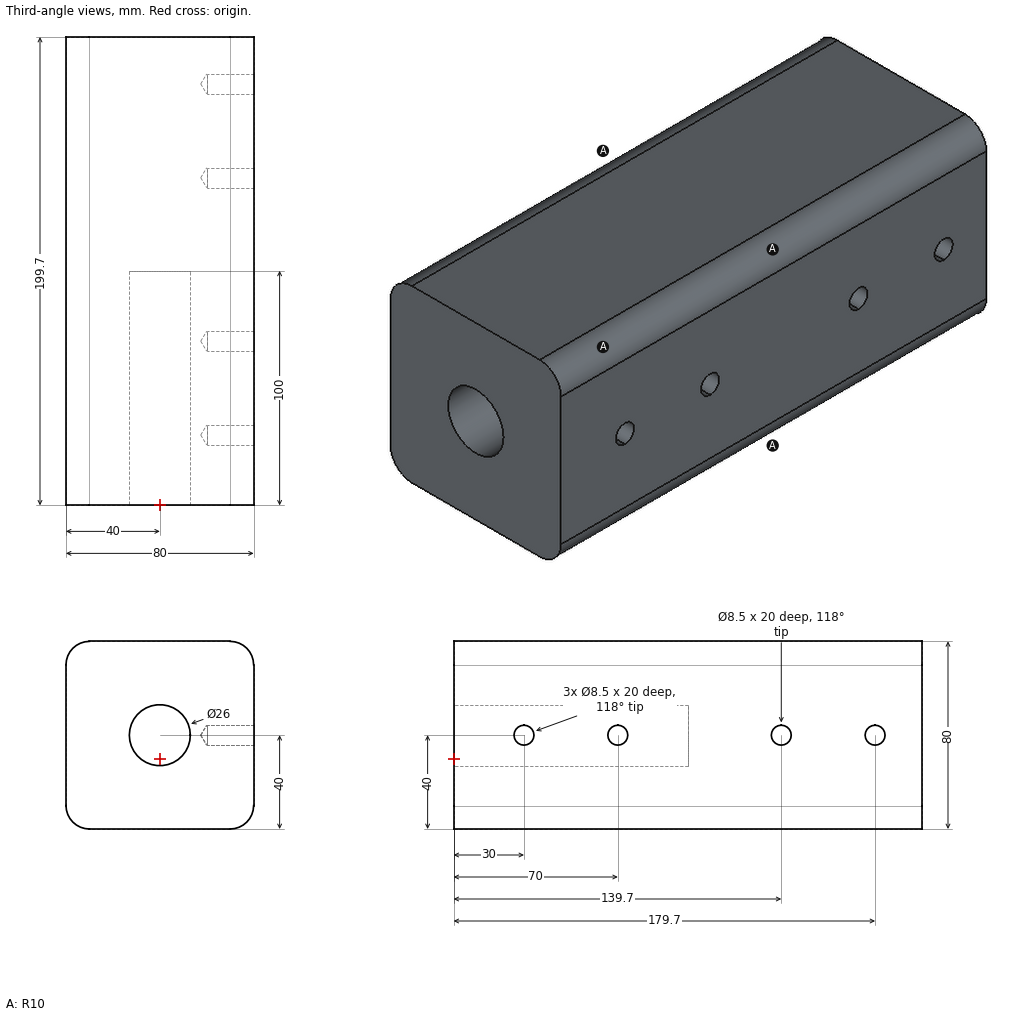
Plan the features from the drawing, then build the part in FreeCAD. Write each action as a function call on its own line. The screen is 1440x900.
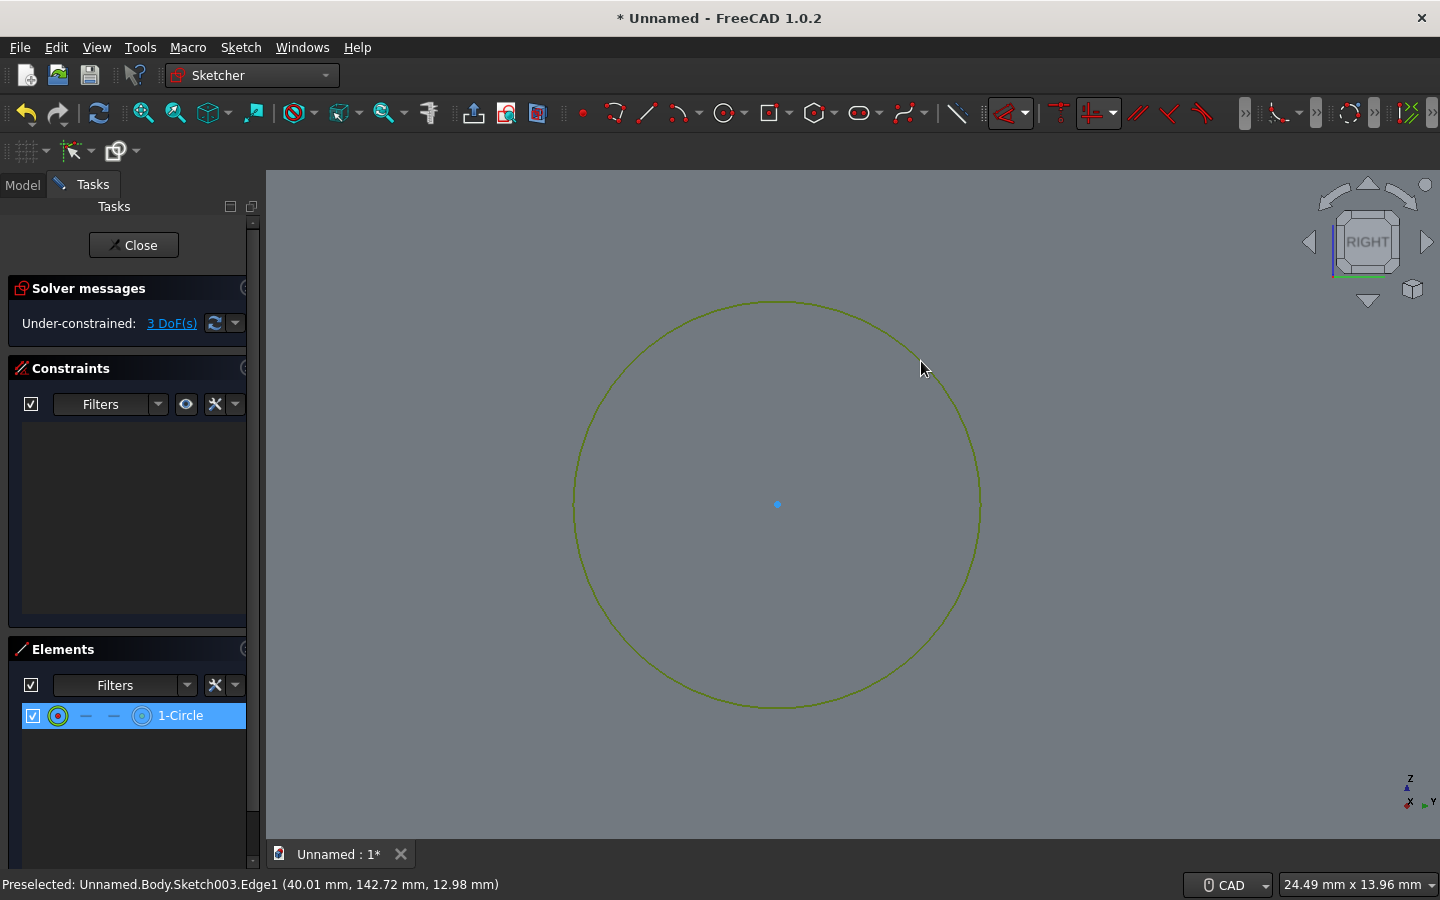
key(k)
key(o)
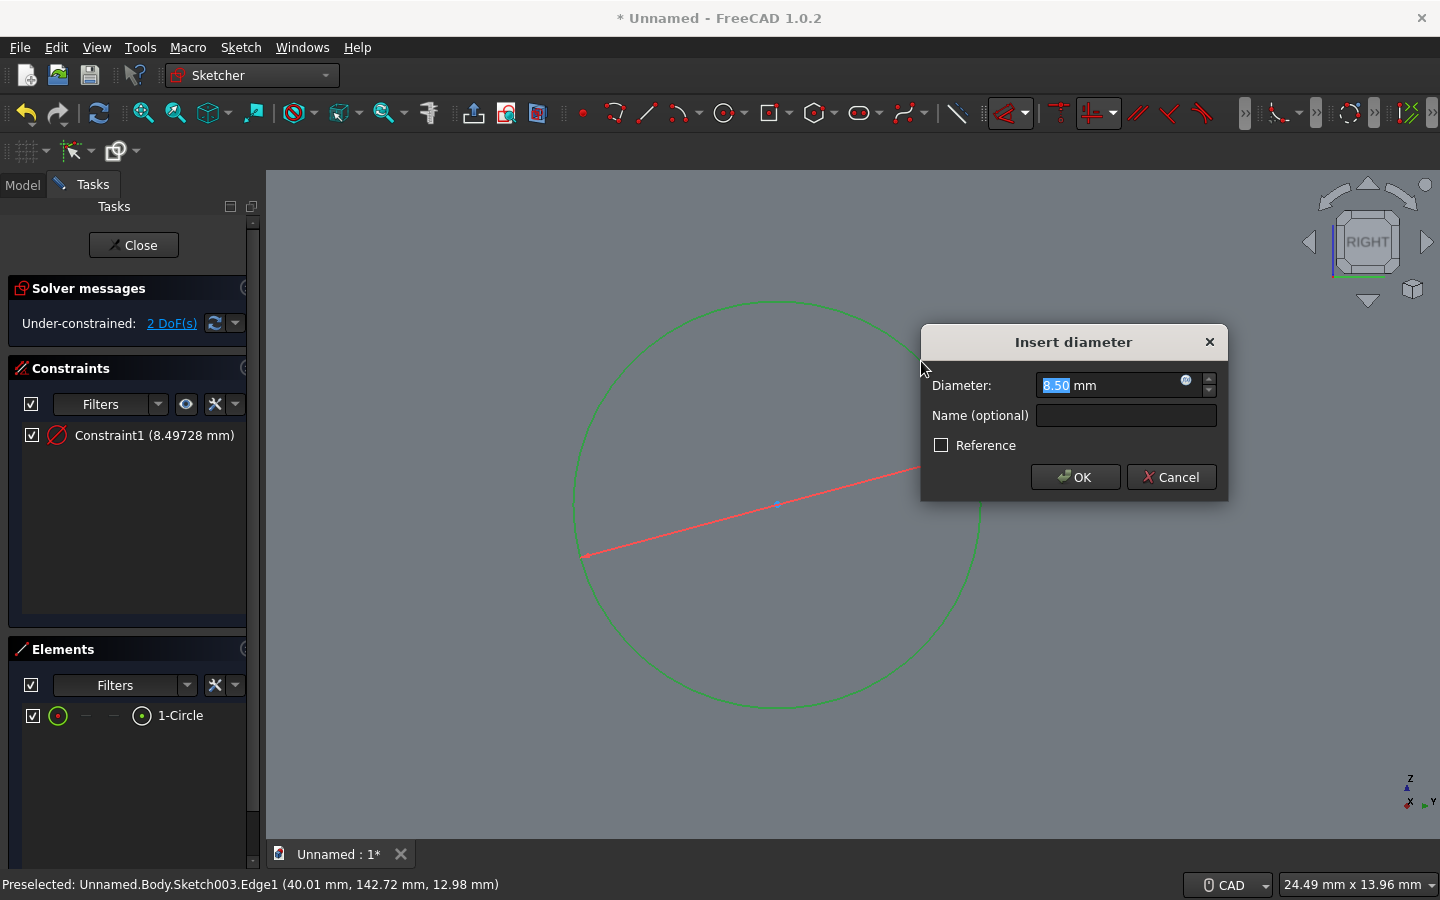
text(8.5)
key(Return)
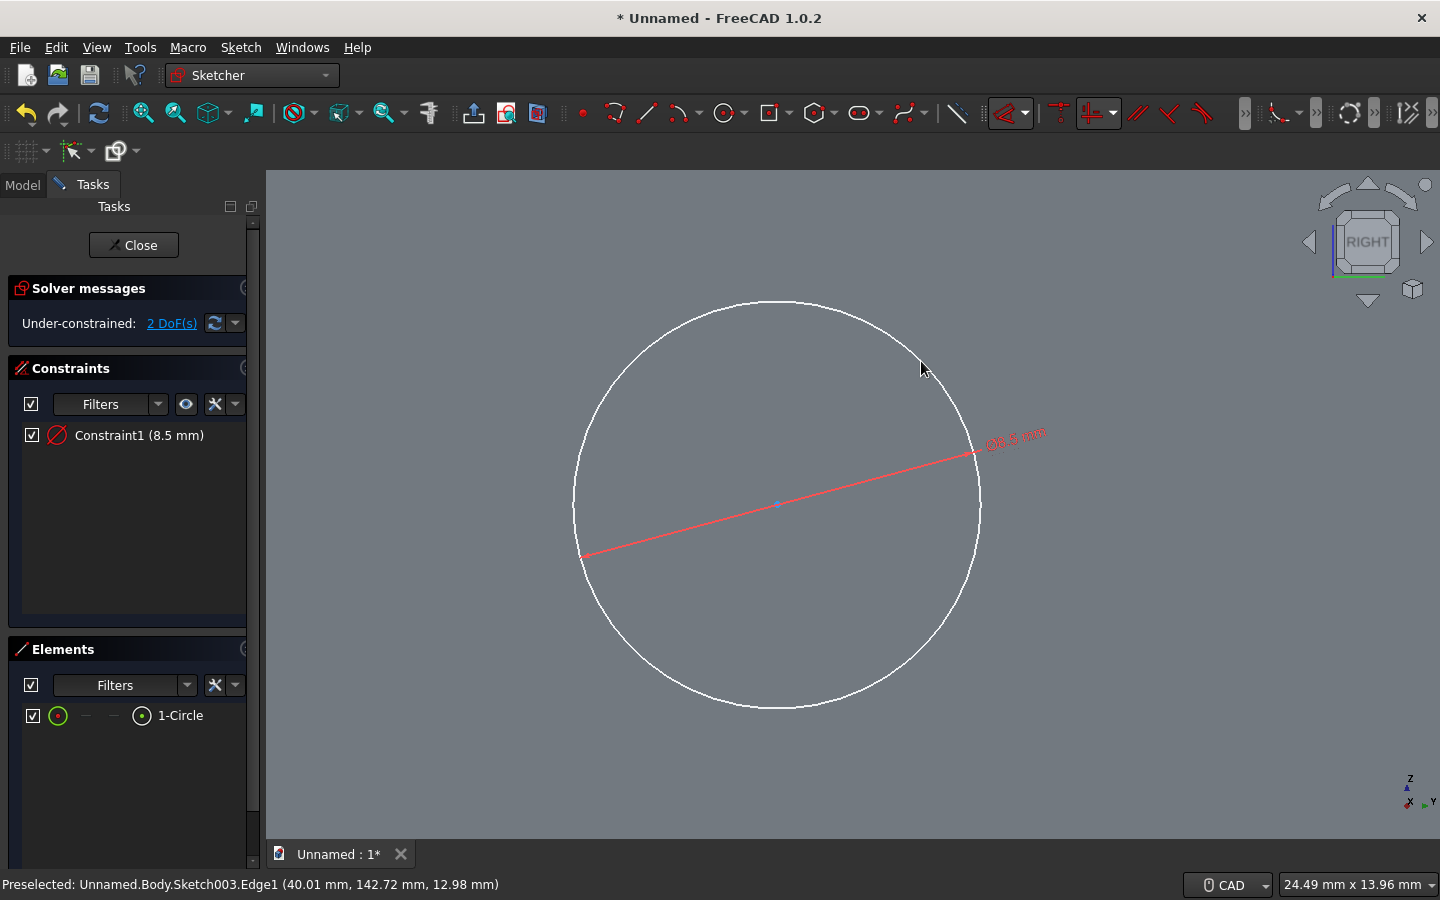
click(777, 505)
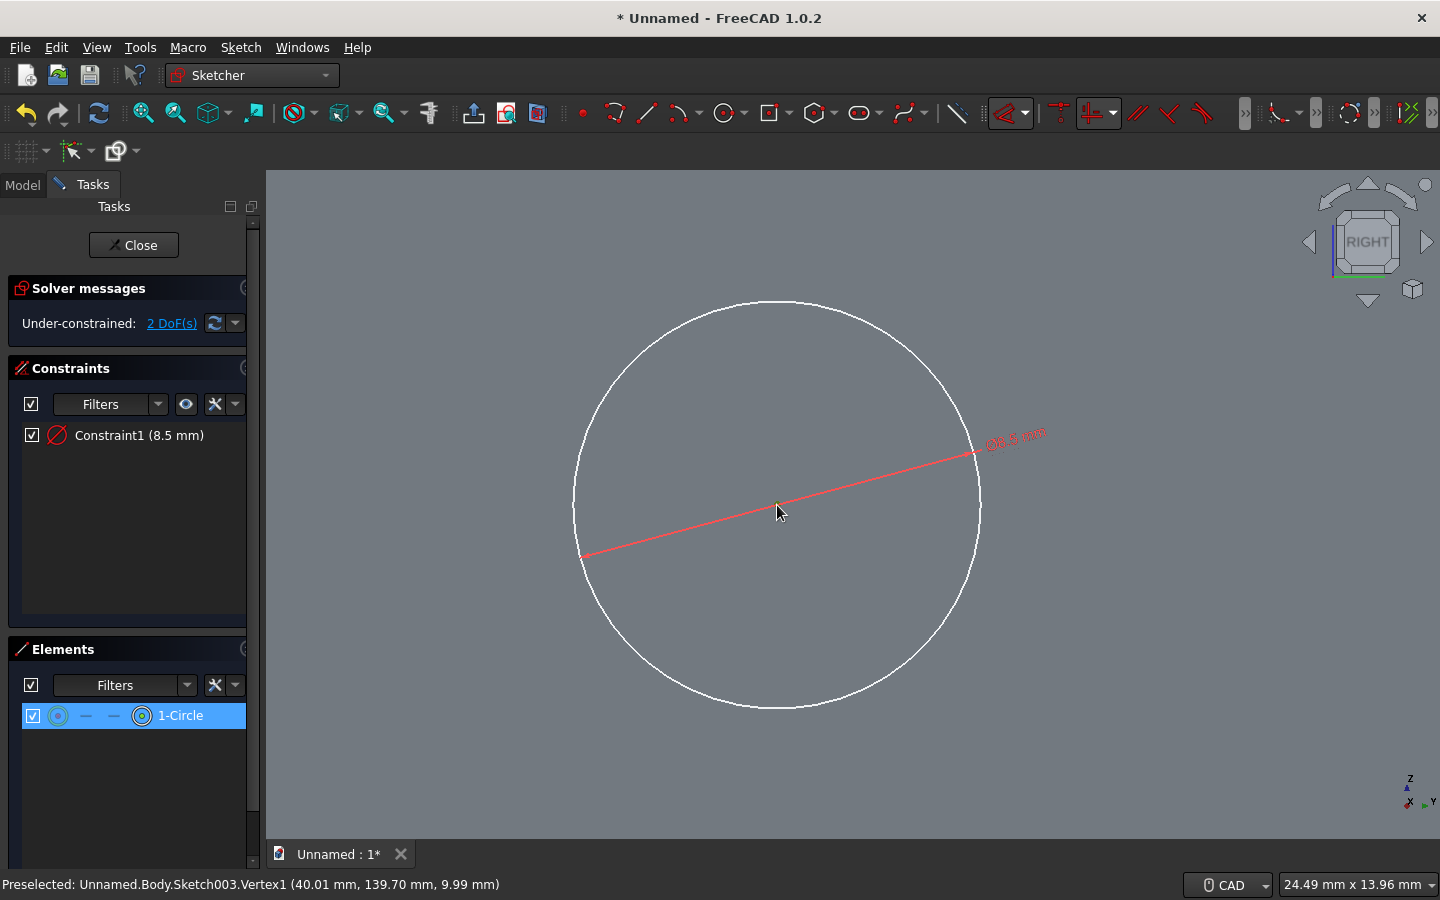
click(1028, 114)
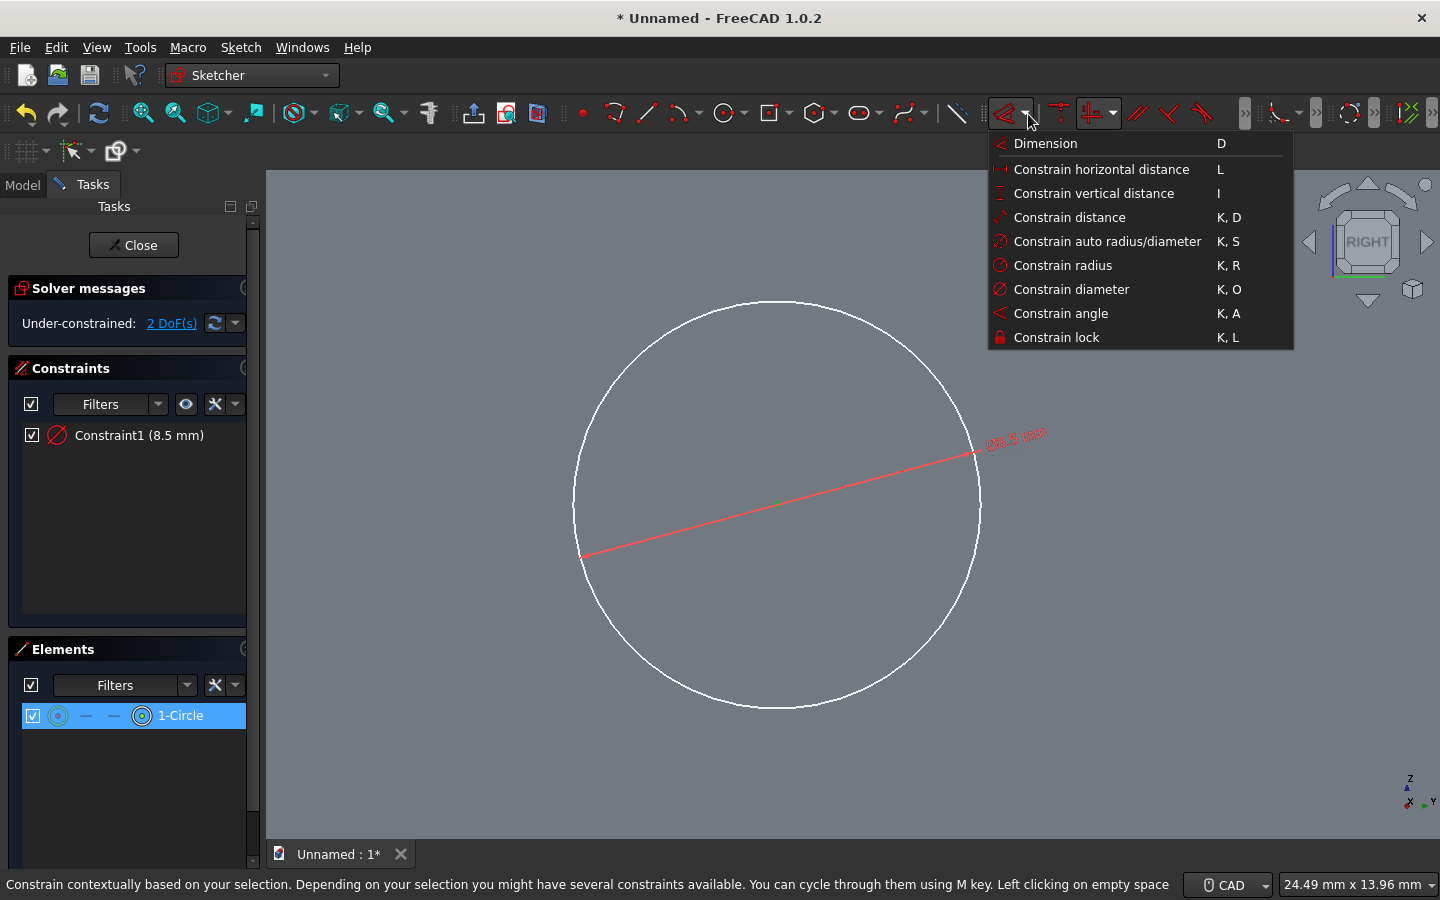
click(1141, 193)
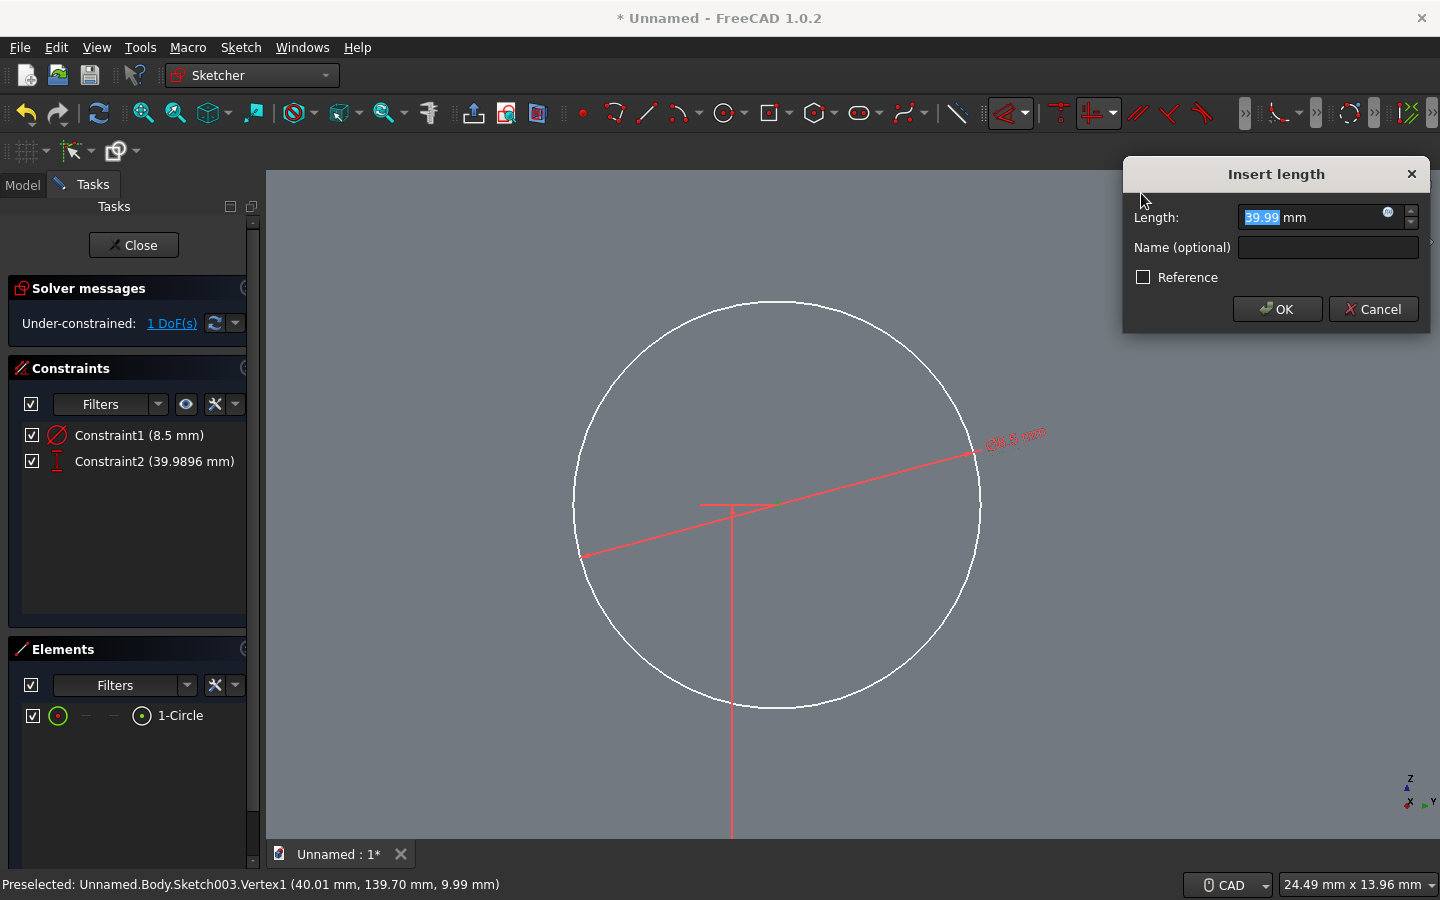
text(40)
key(Return)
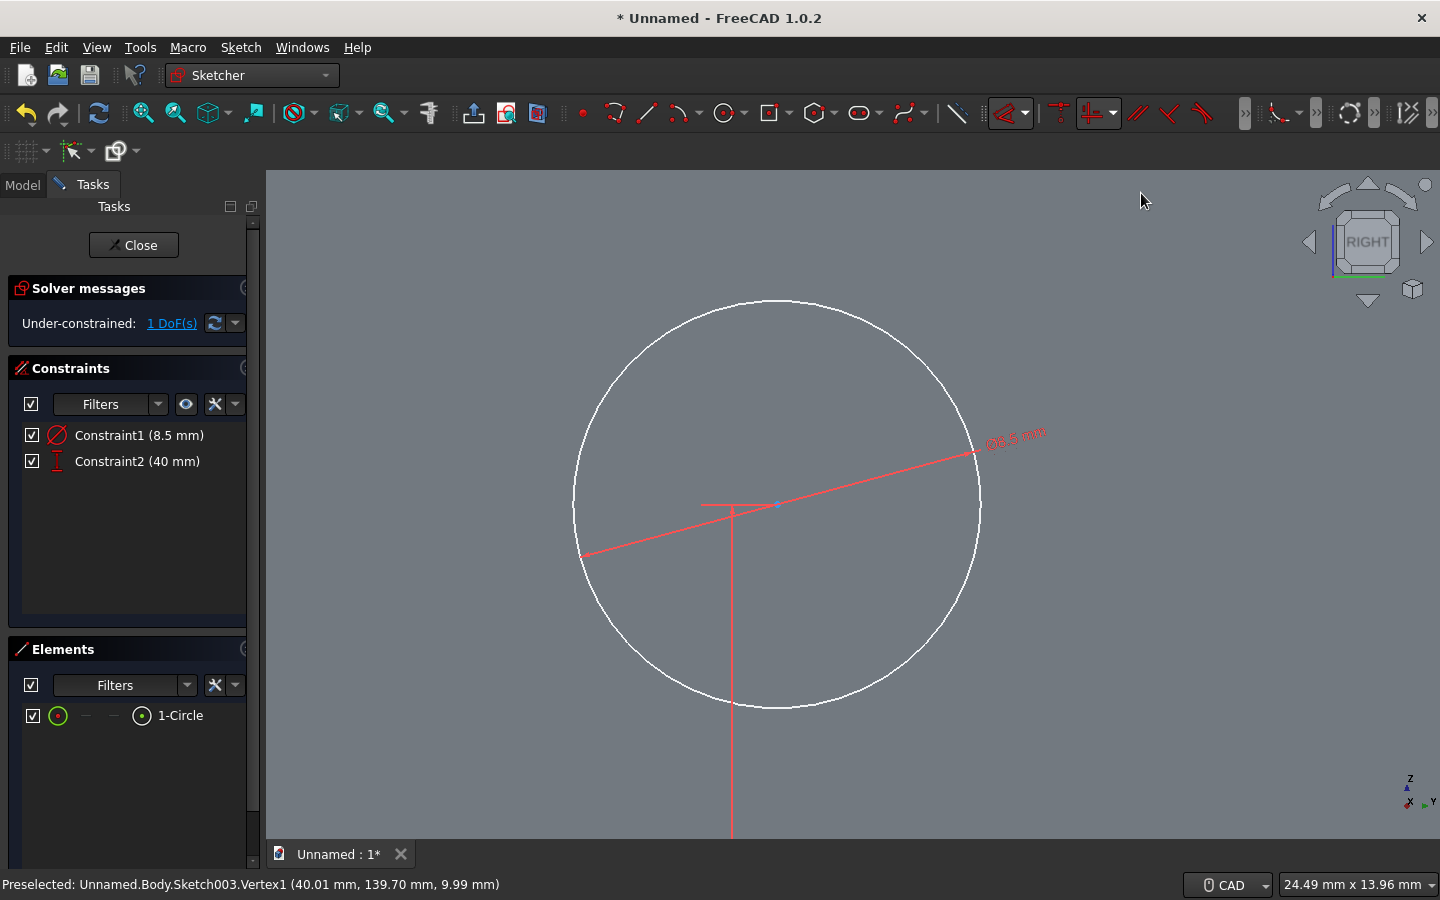
click(777, 504)